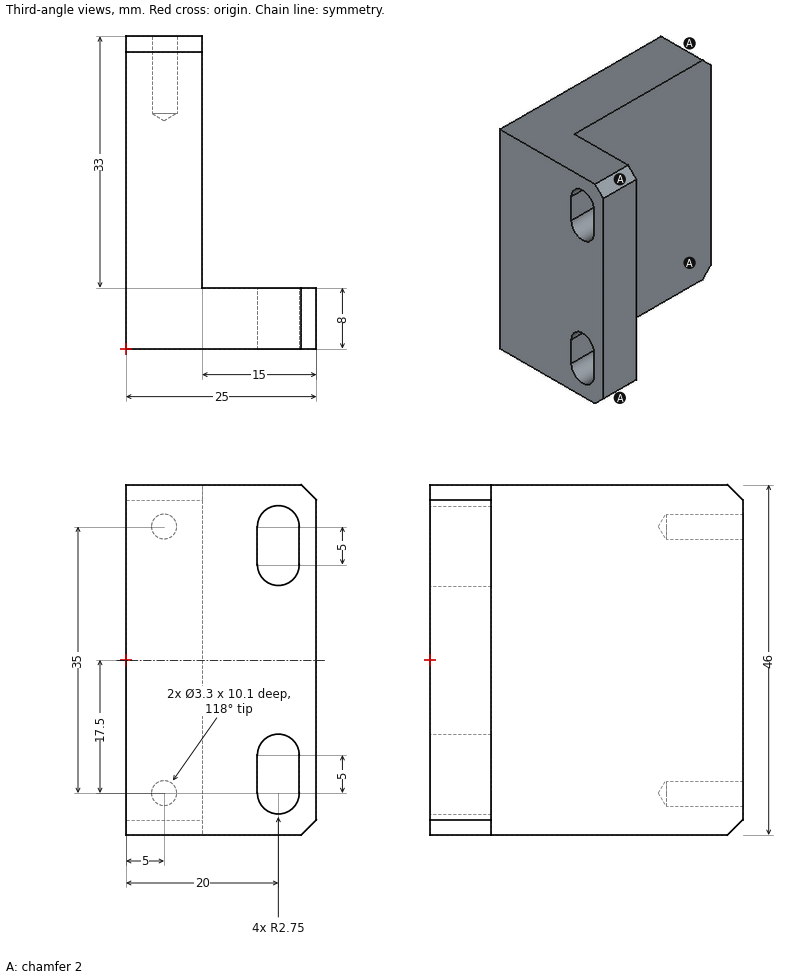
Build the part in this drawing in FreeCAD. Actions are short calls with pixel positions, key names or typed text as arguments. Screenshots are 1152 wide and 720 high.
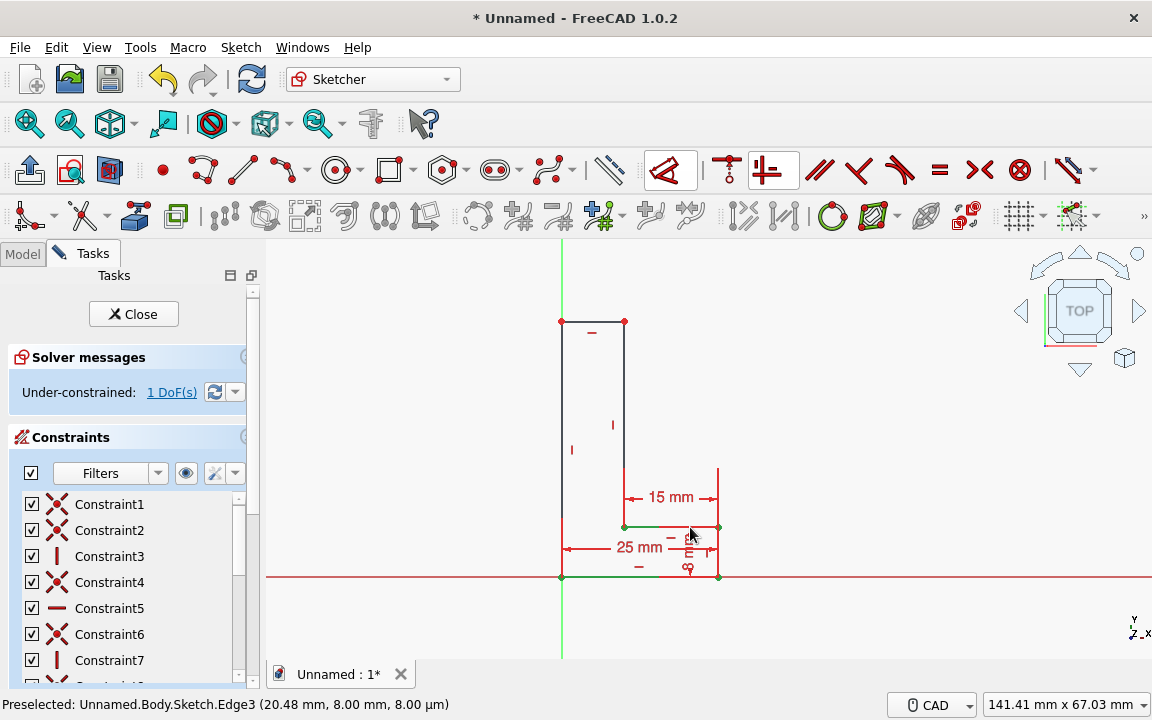
click(624, 466)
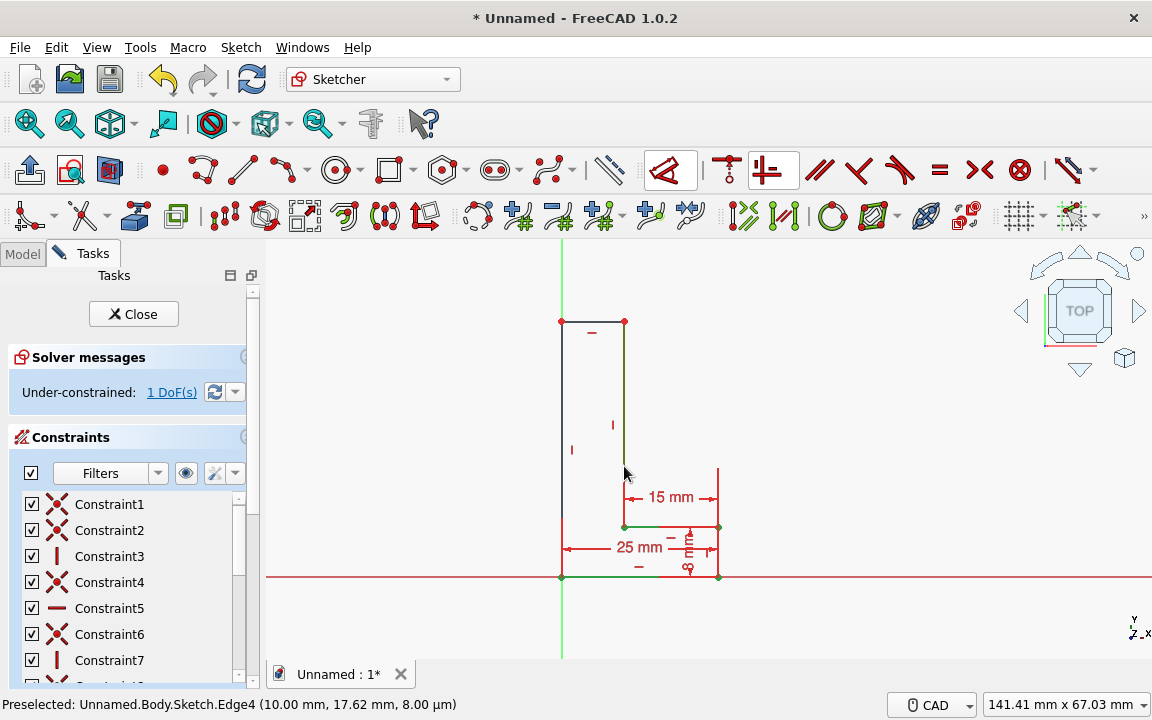
click(692, 170)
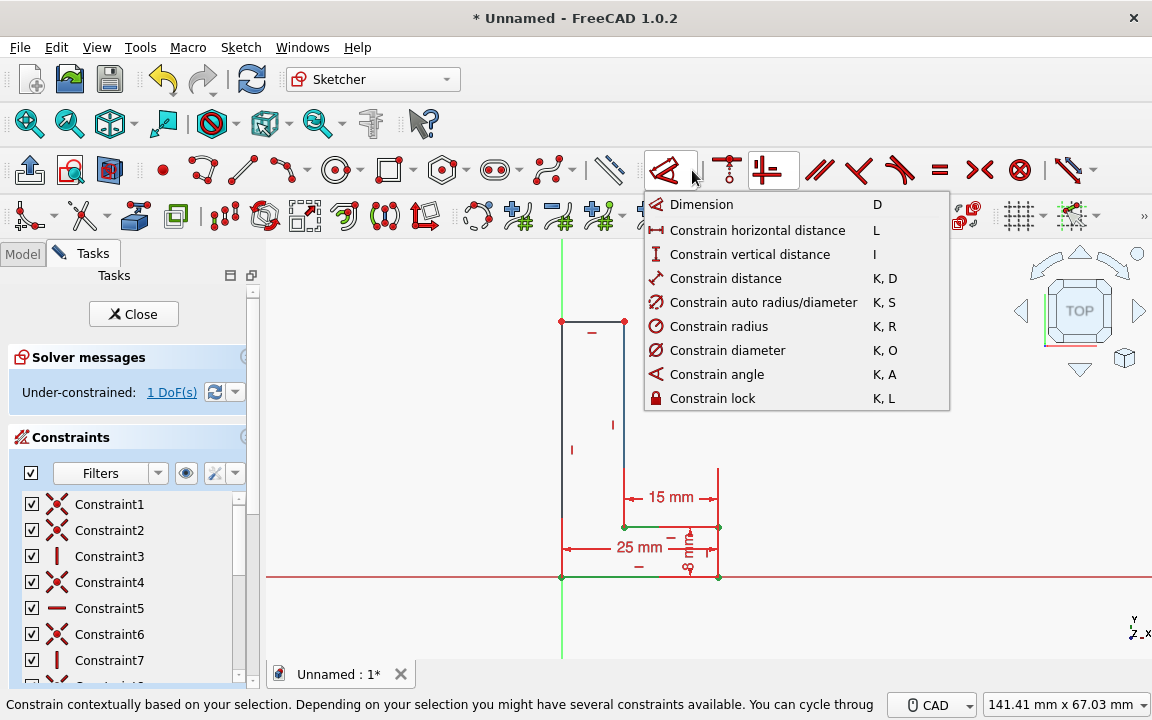
click(797, 254)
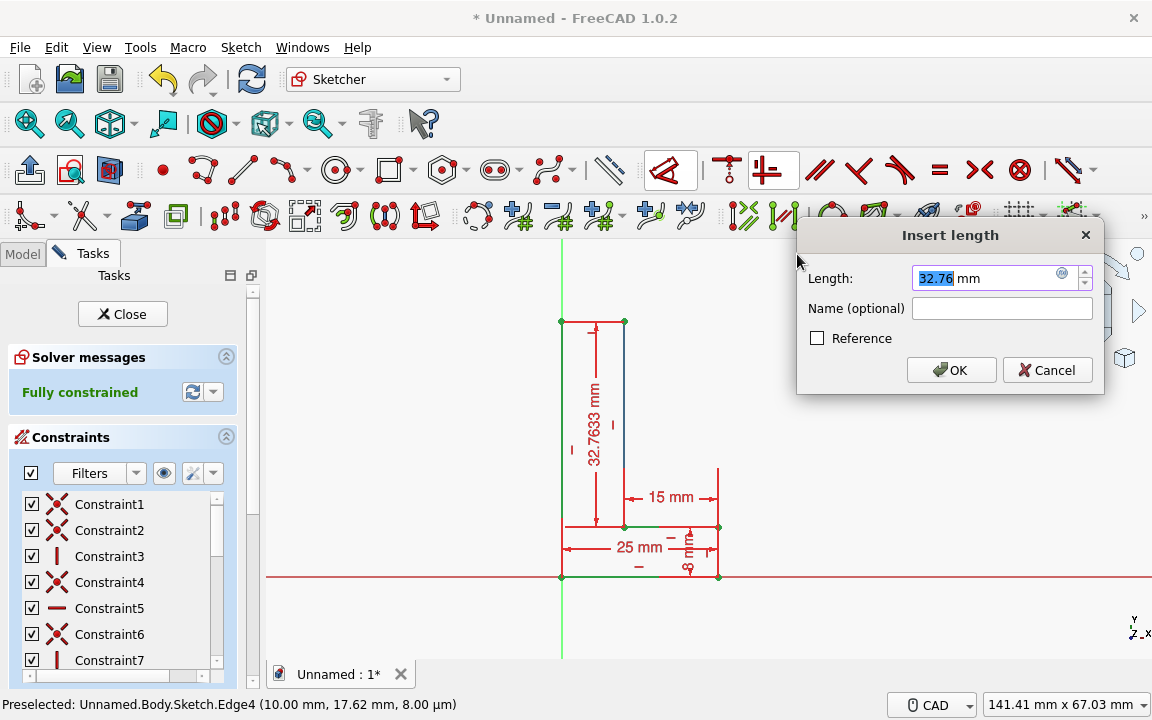
text(33)
key(Return)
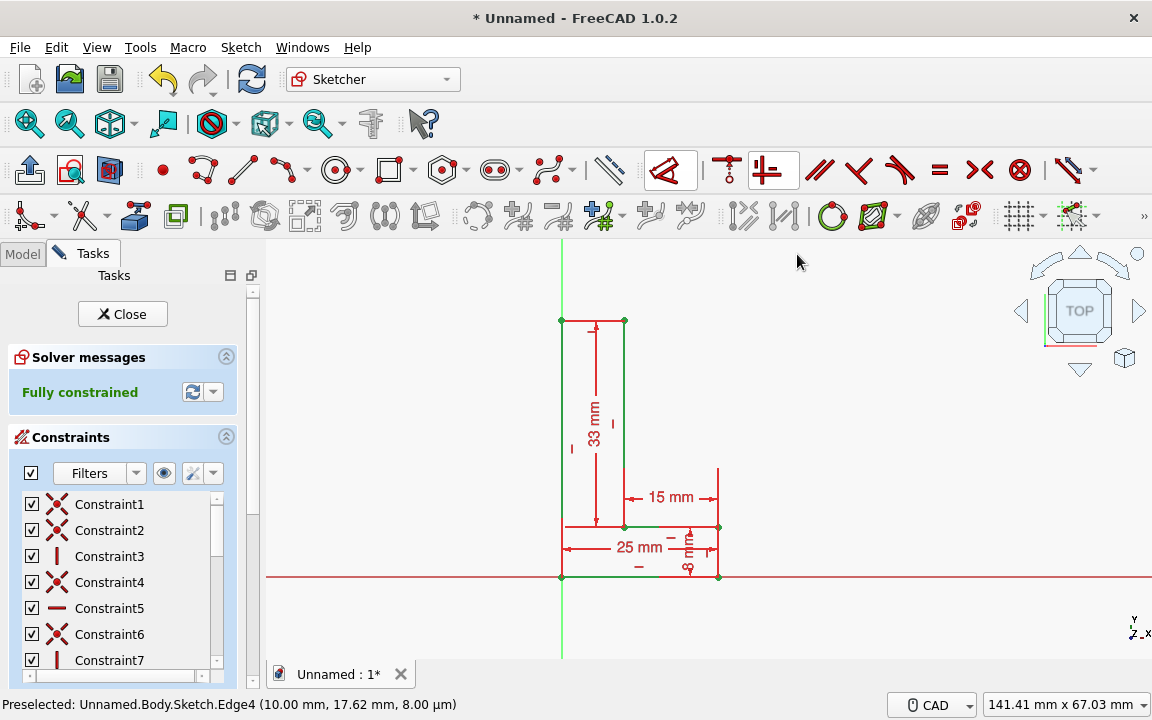
click(123, 314)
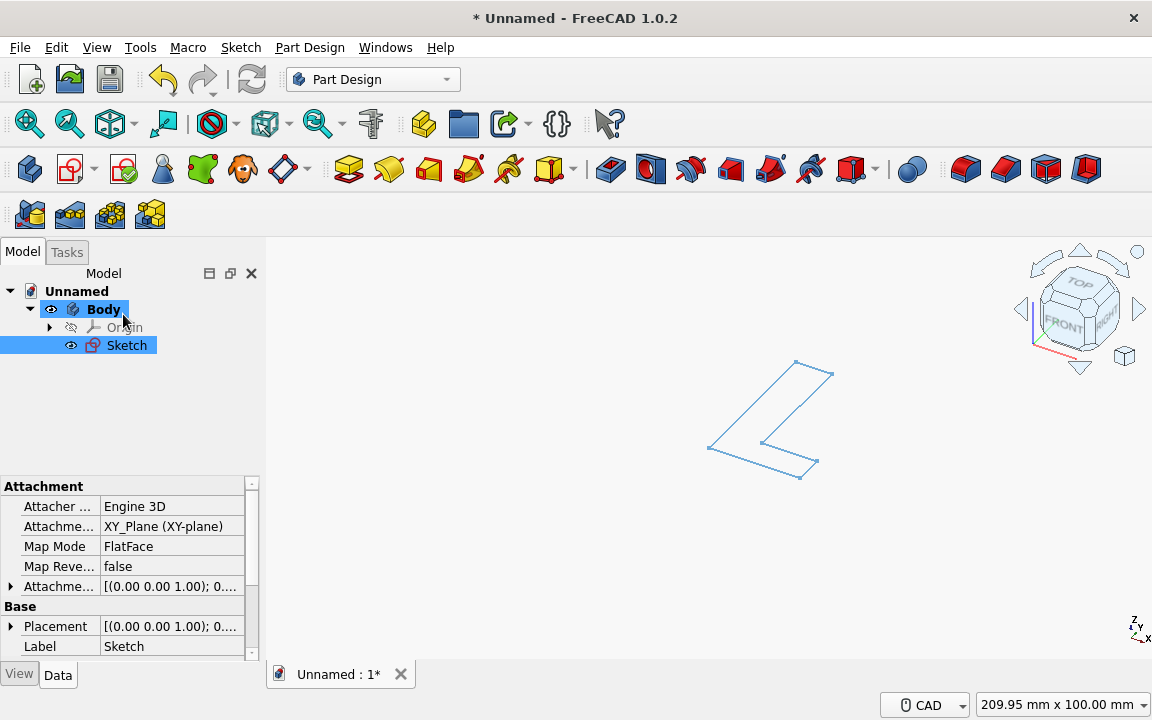
click(350, 170)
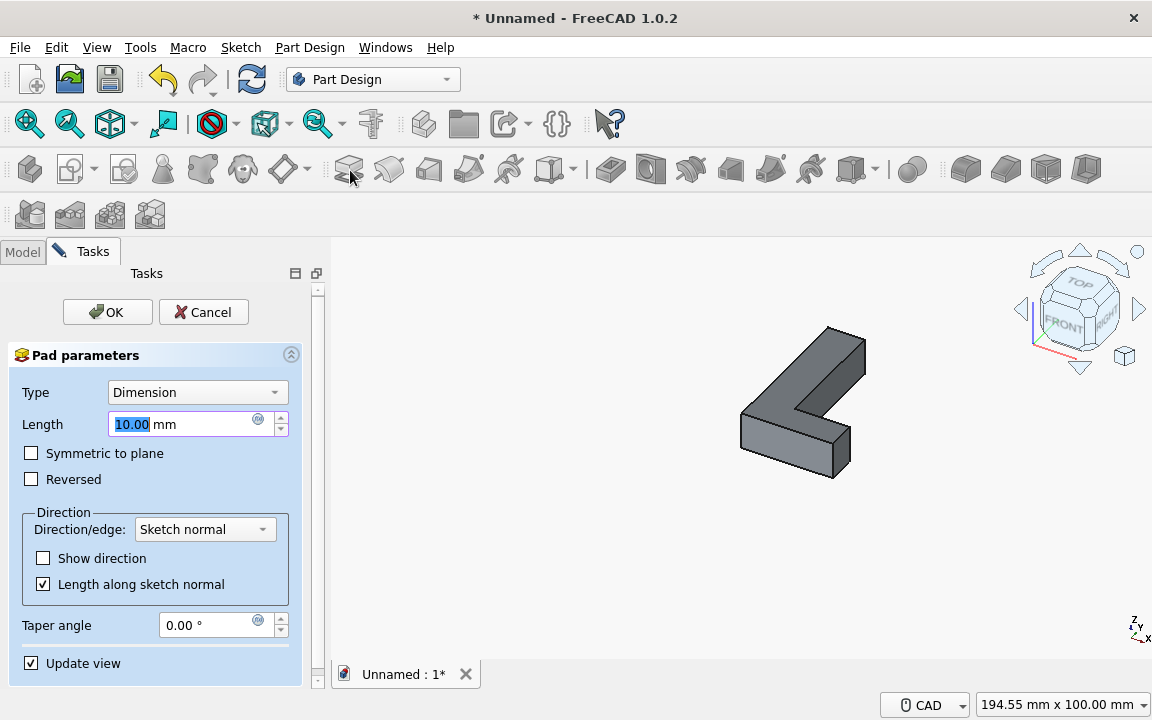
text(46)
key(Tab)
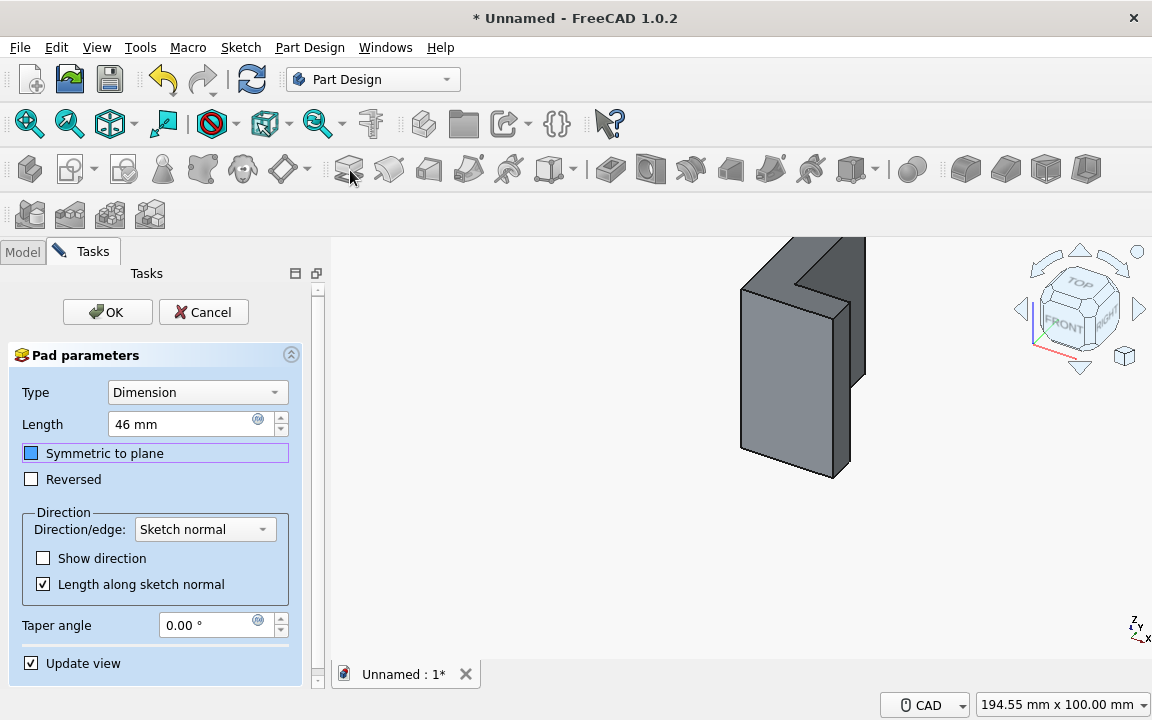
click(30, 453)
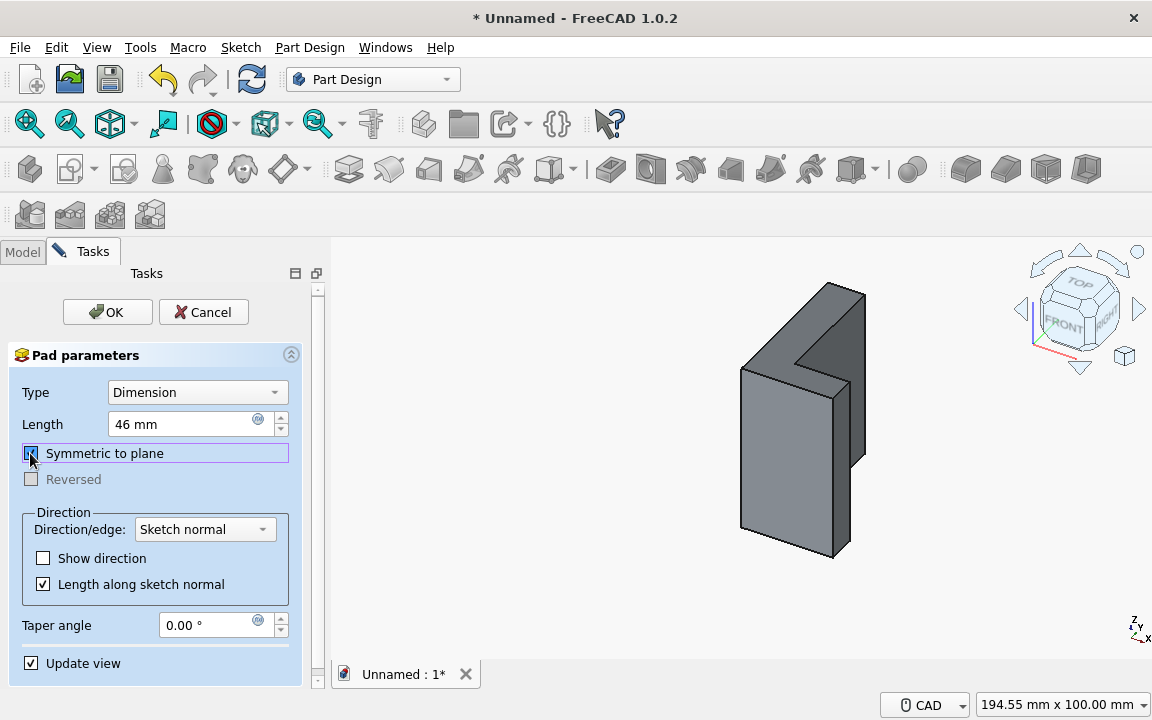
click(108, 312)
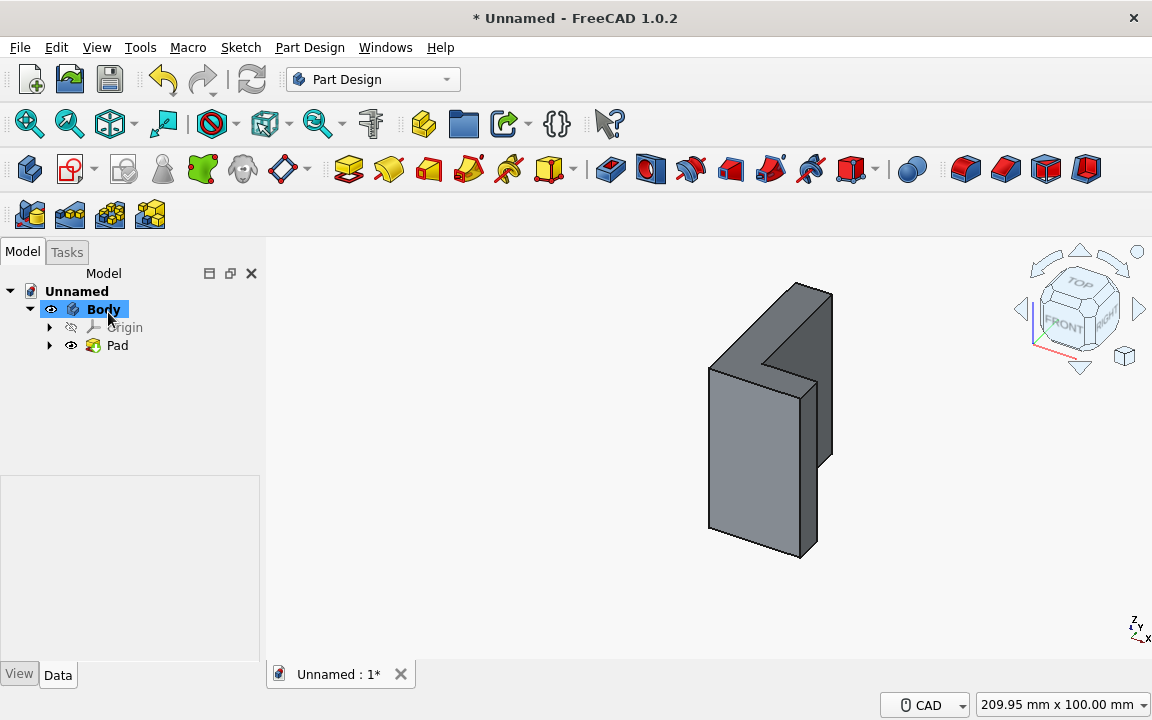
click(70, 170)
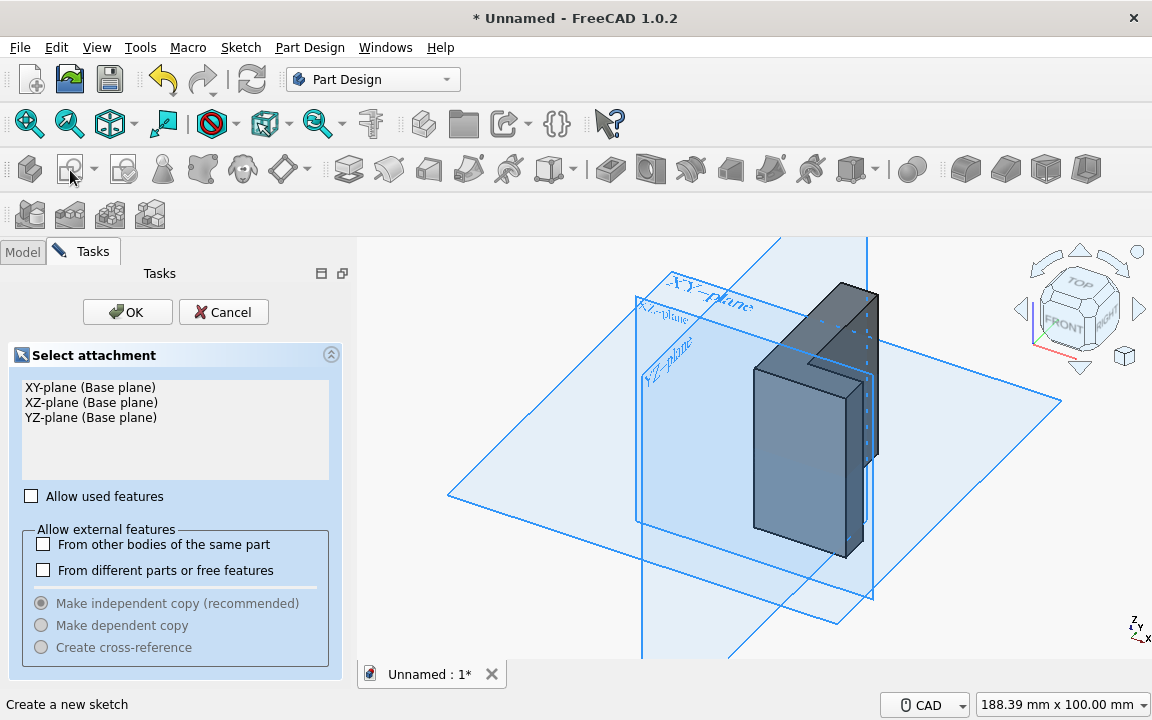
click(82, 402)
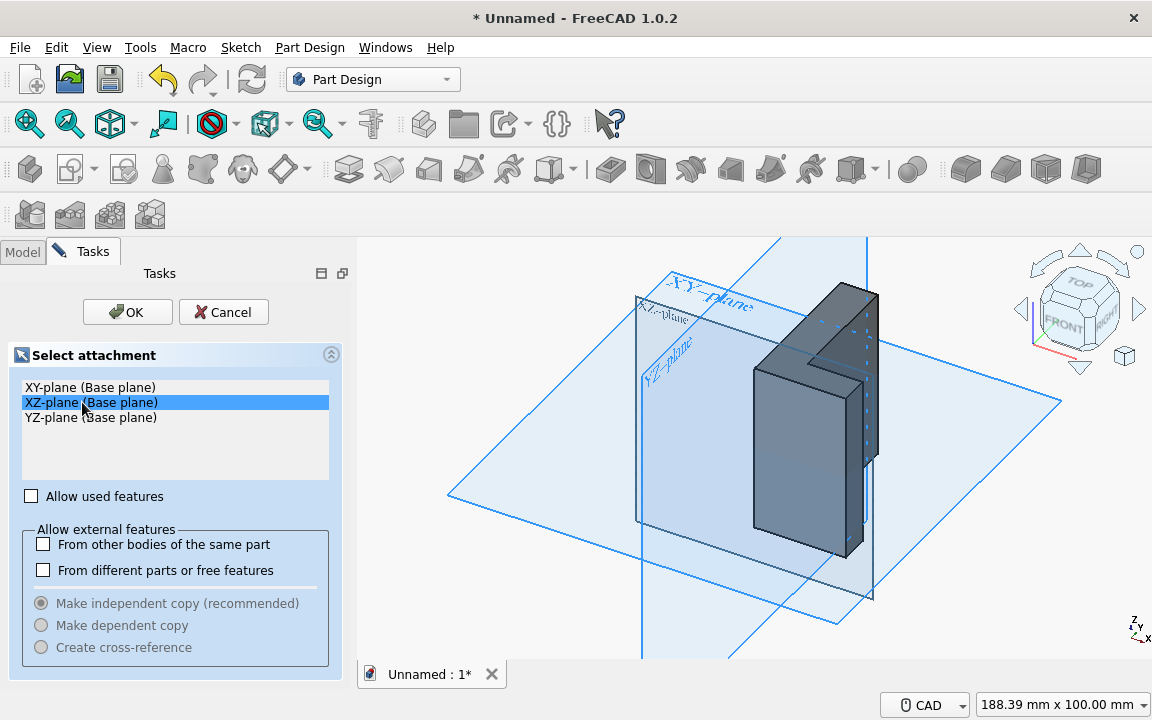
click(128, 312)